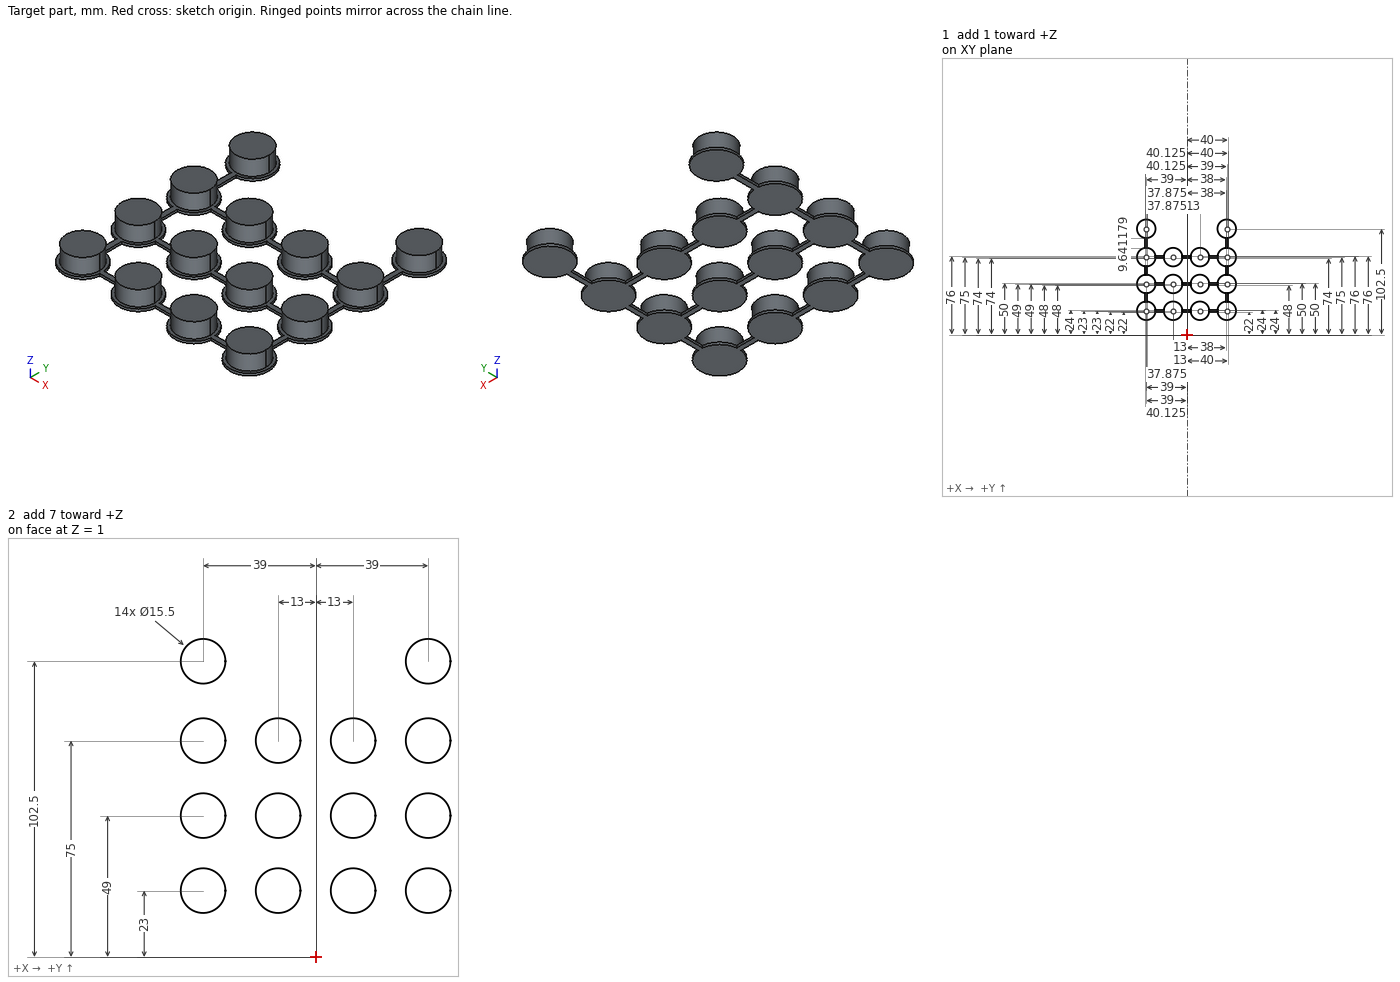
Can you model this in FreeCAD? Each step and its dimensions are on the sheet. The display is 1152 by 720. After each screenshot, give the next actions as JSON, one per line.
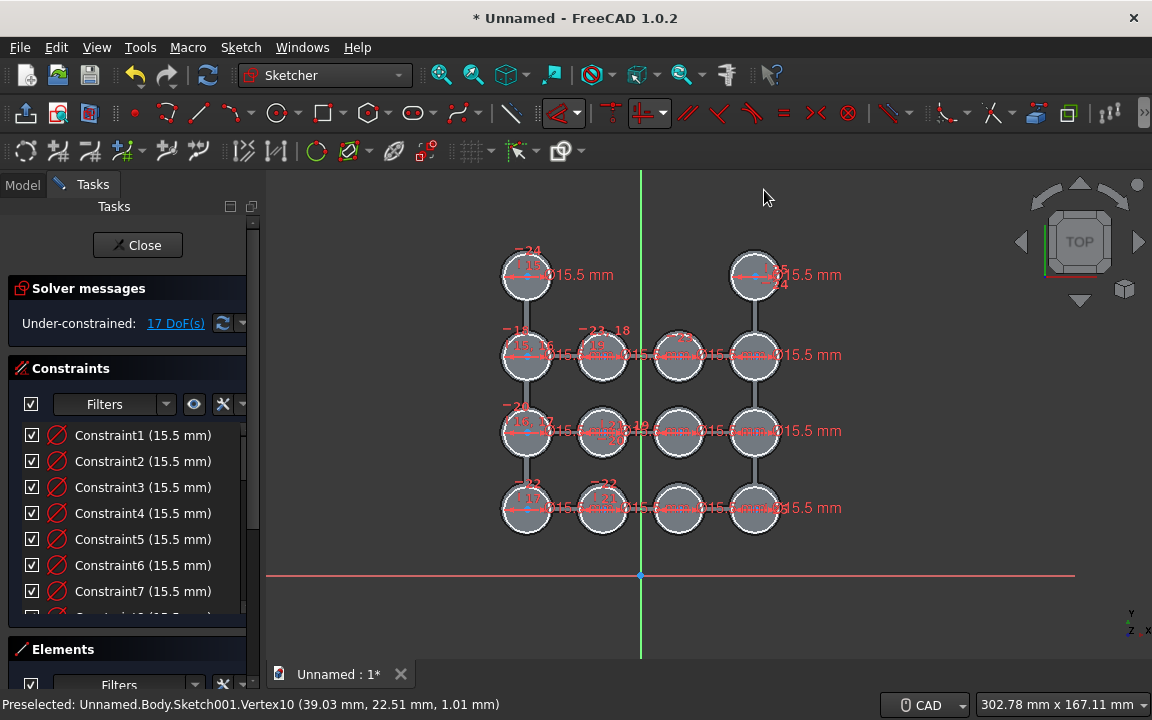
{"action": "left_click", "coordinate": [603, 510]}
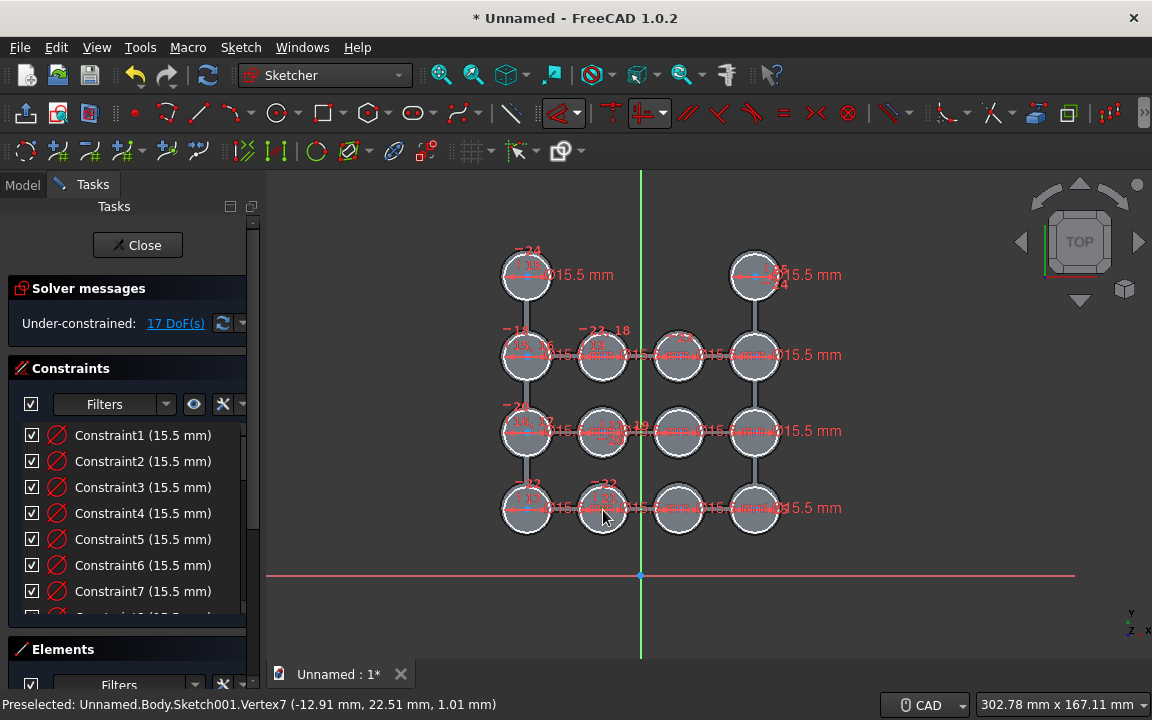
{"action": "left_click", "coordinate": [755, 510]}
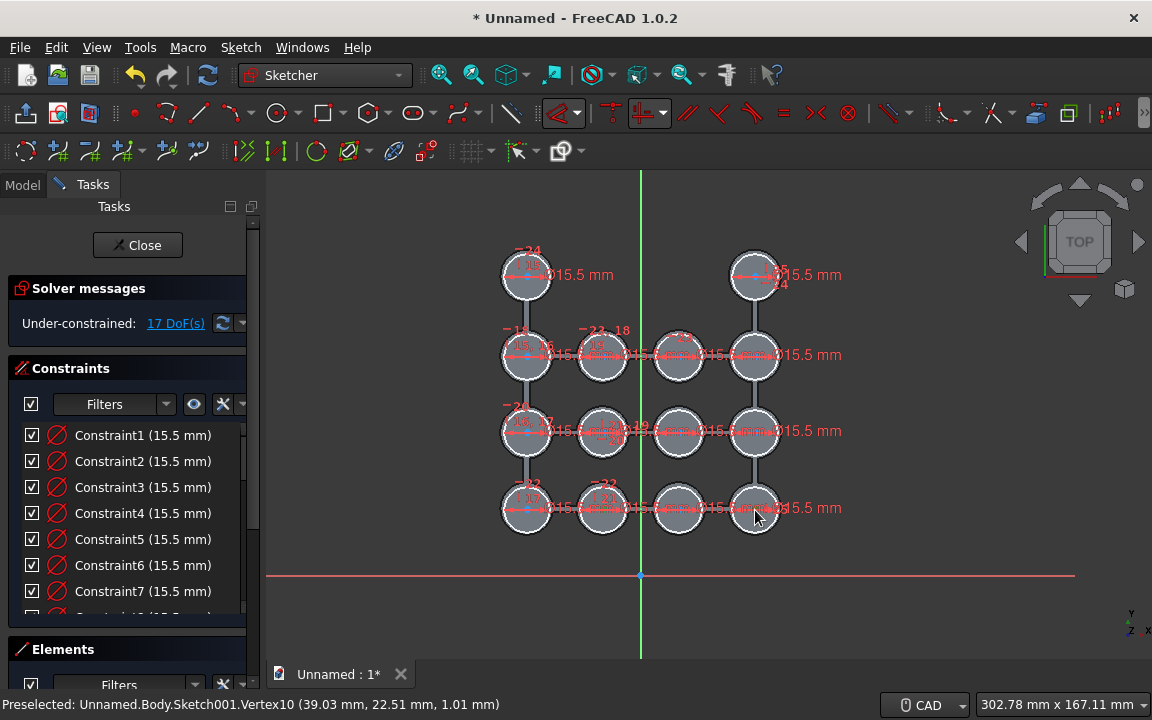
{"action": "left_click", "coordinate": [666, 114]}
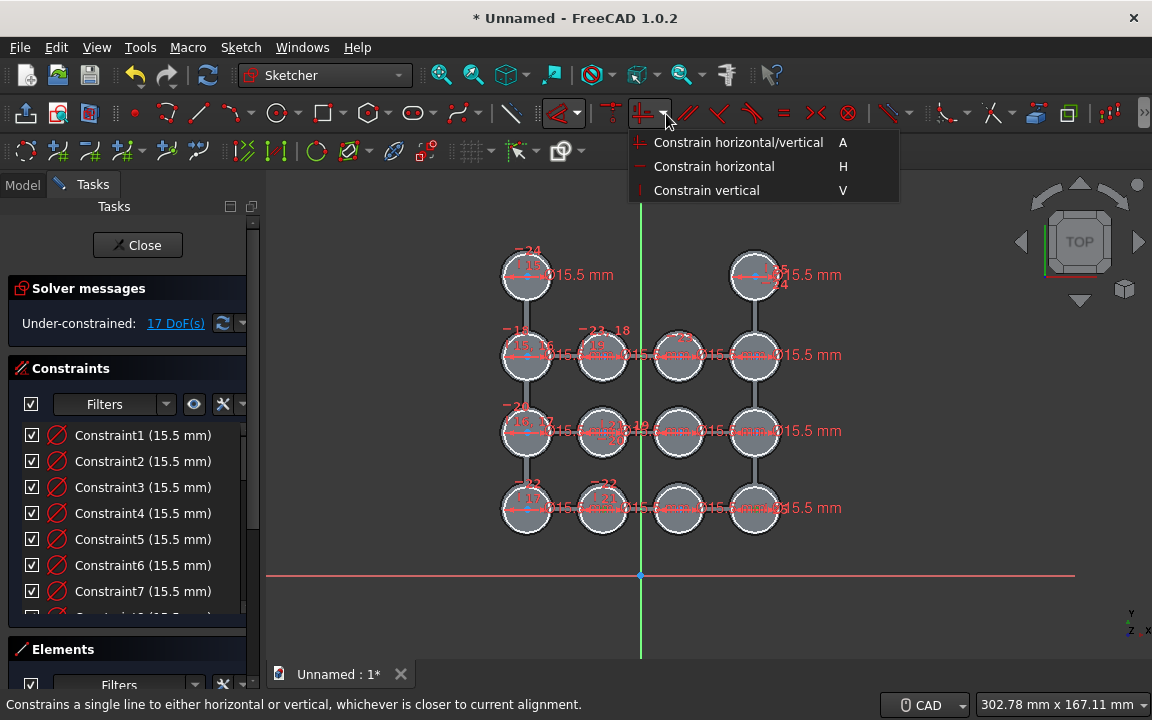
{"action": "left_click", "coordinate": [764, 166]}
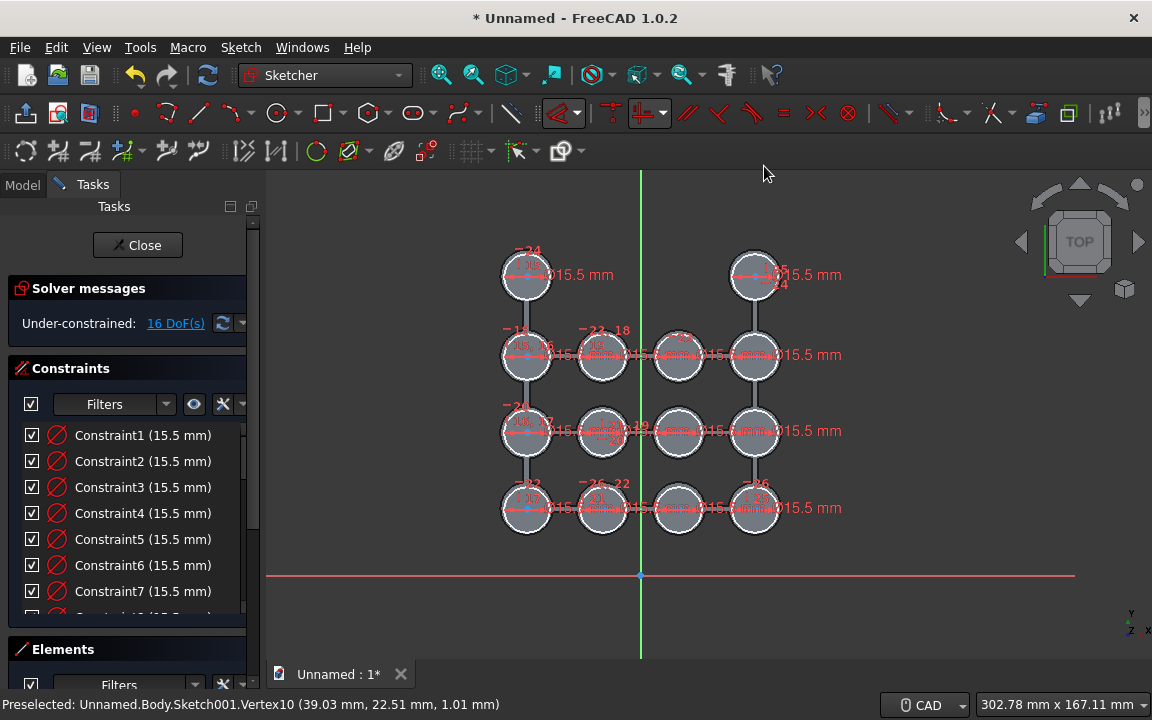
{"action": "left_click", "coordinate": [679, 357]}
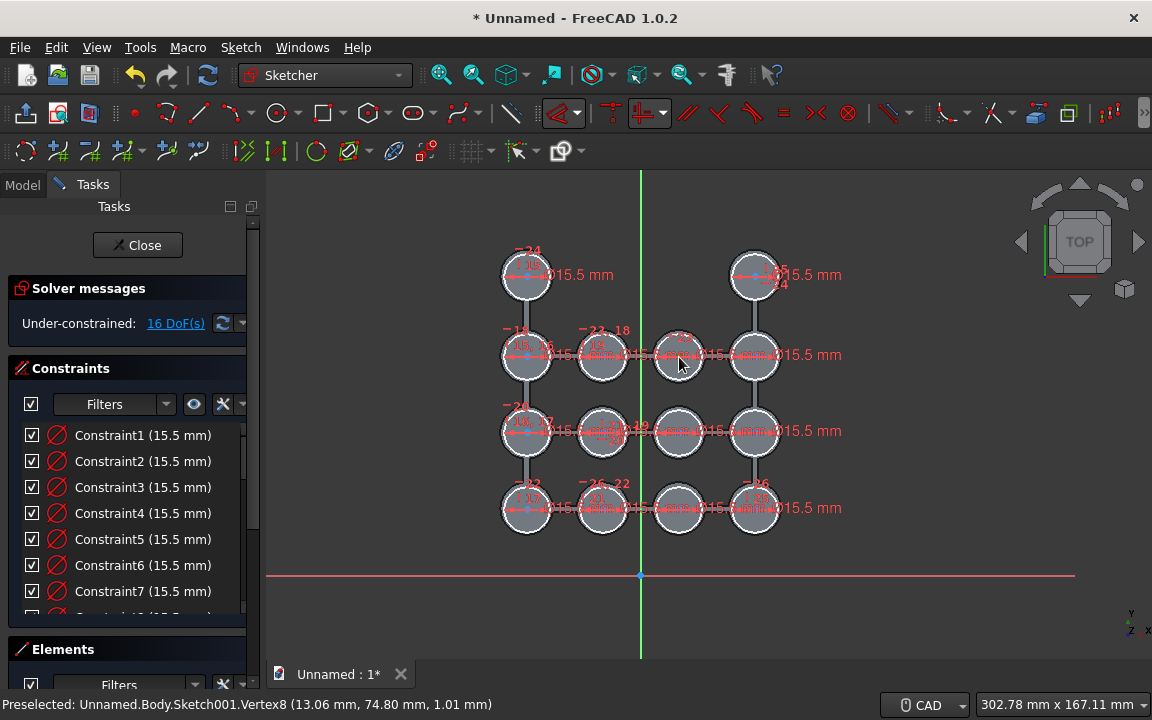
{"action": "left_click", "coordinate": [679, 510]}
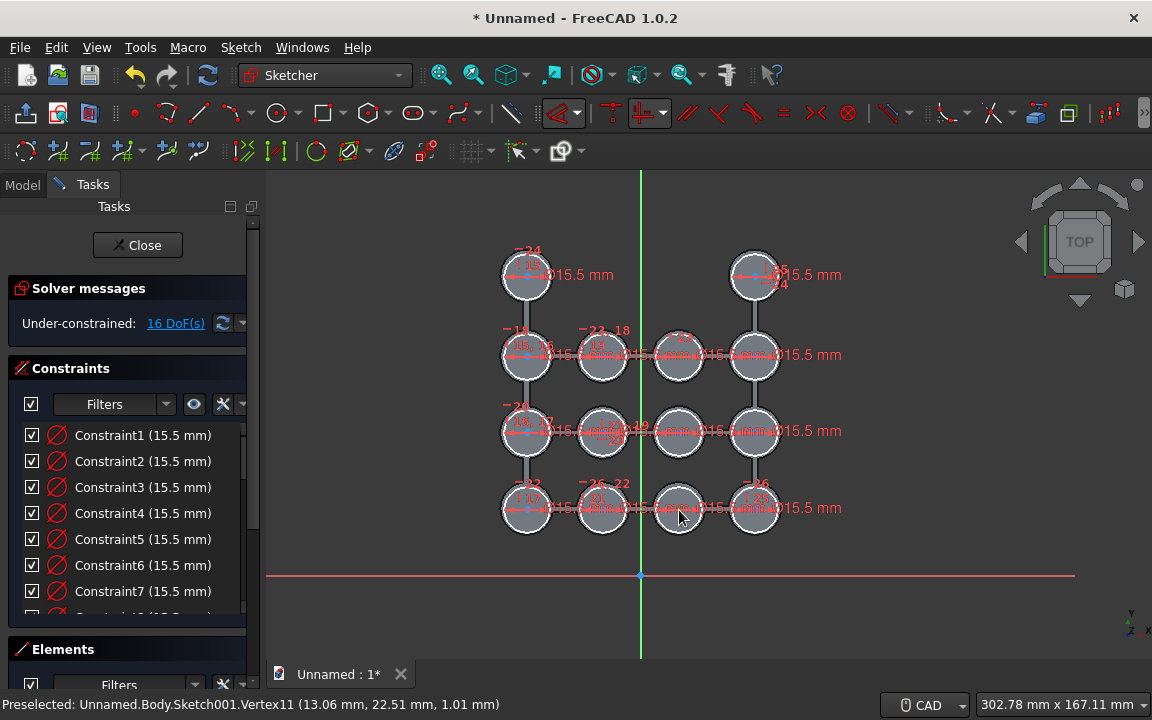
{"action": "left_click", "coordinate": [666, 114]}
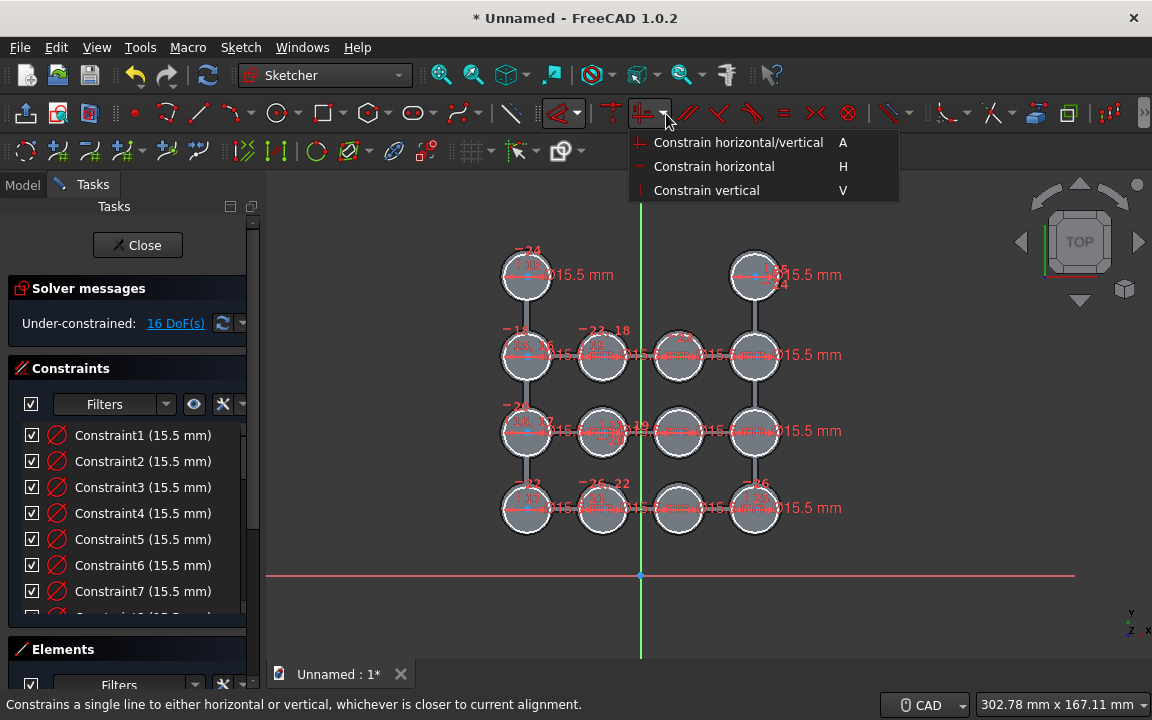
{"action": "left_click", "coordinate": [764, 190]}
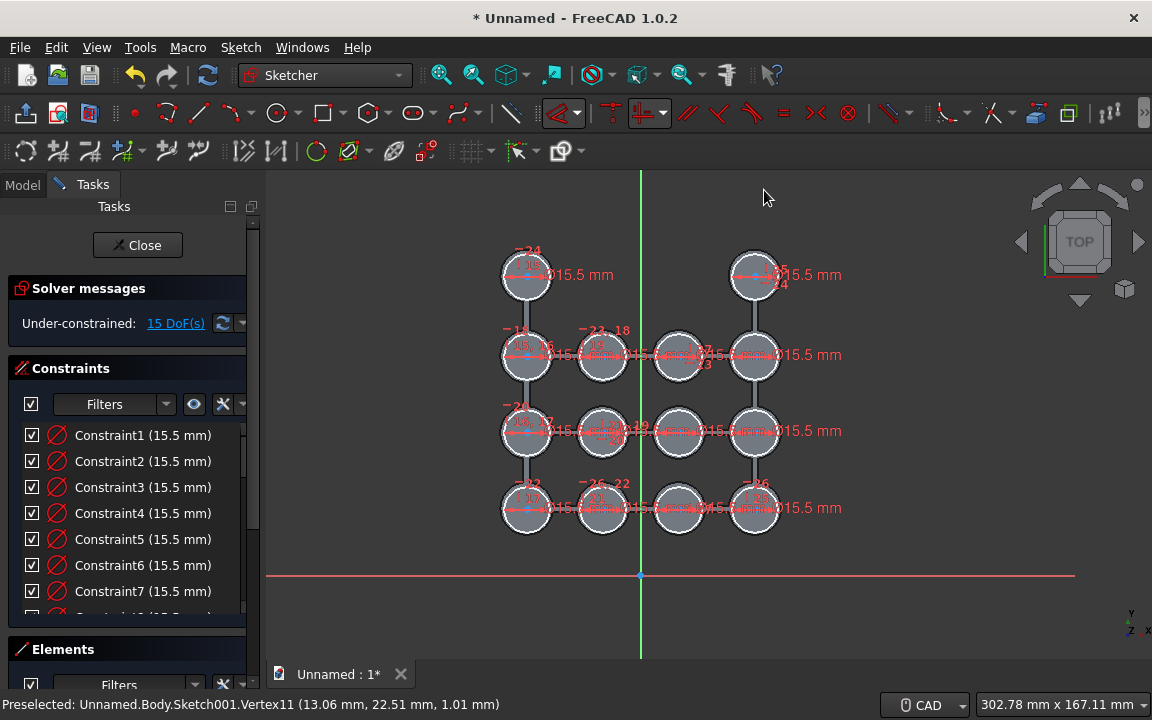
{"action": "left_click", "coordinate": [603, 510]}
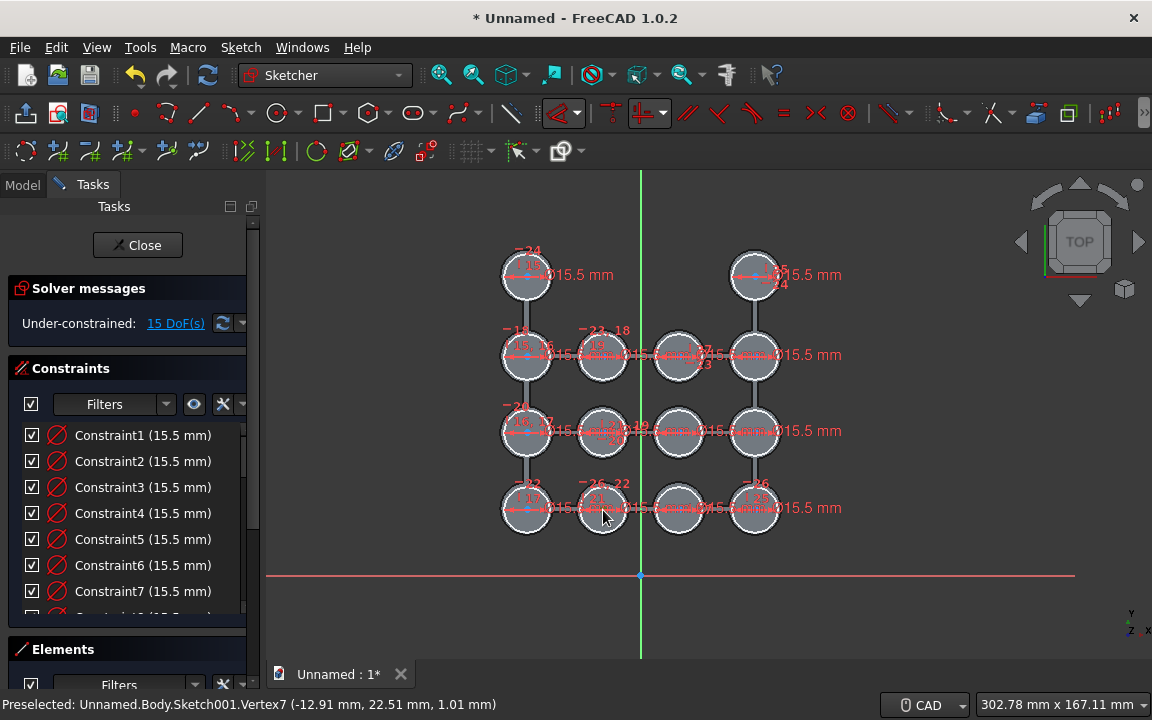
{"action": "left_click", "coordinate": [679, 510]}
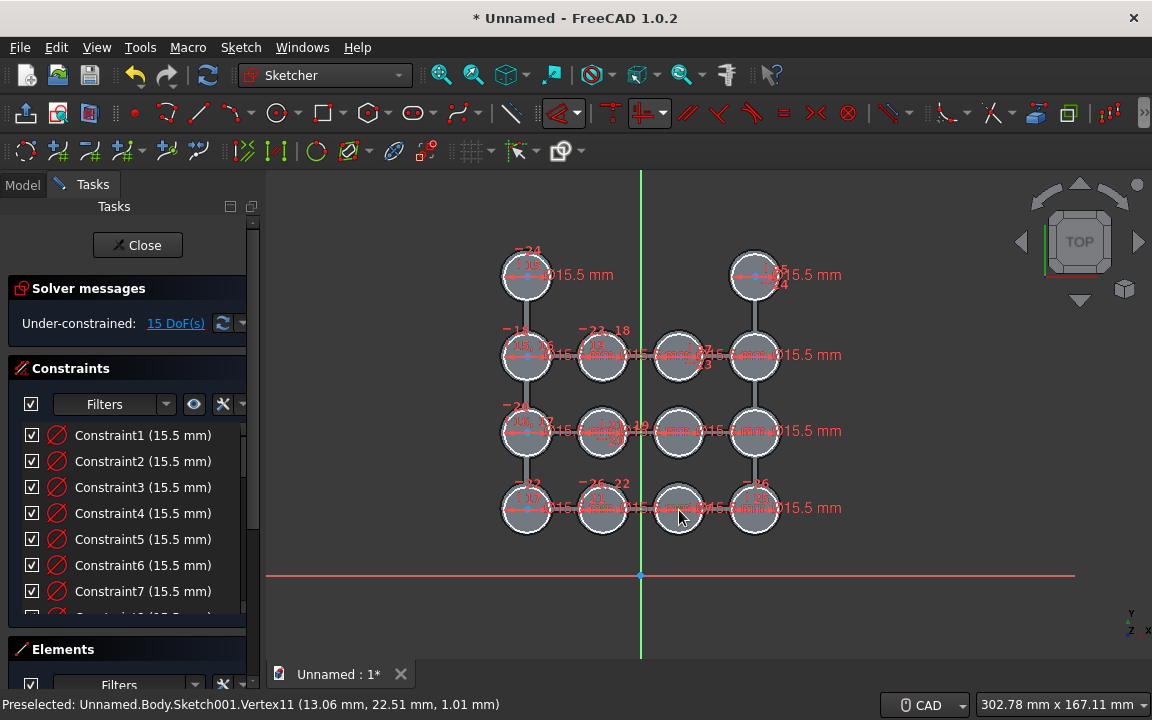
{"action": "left_click", "coordinate": [666, 114]}